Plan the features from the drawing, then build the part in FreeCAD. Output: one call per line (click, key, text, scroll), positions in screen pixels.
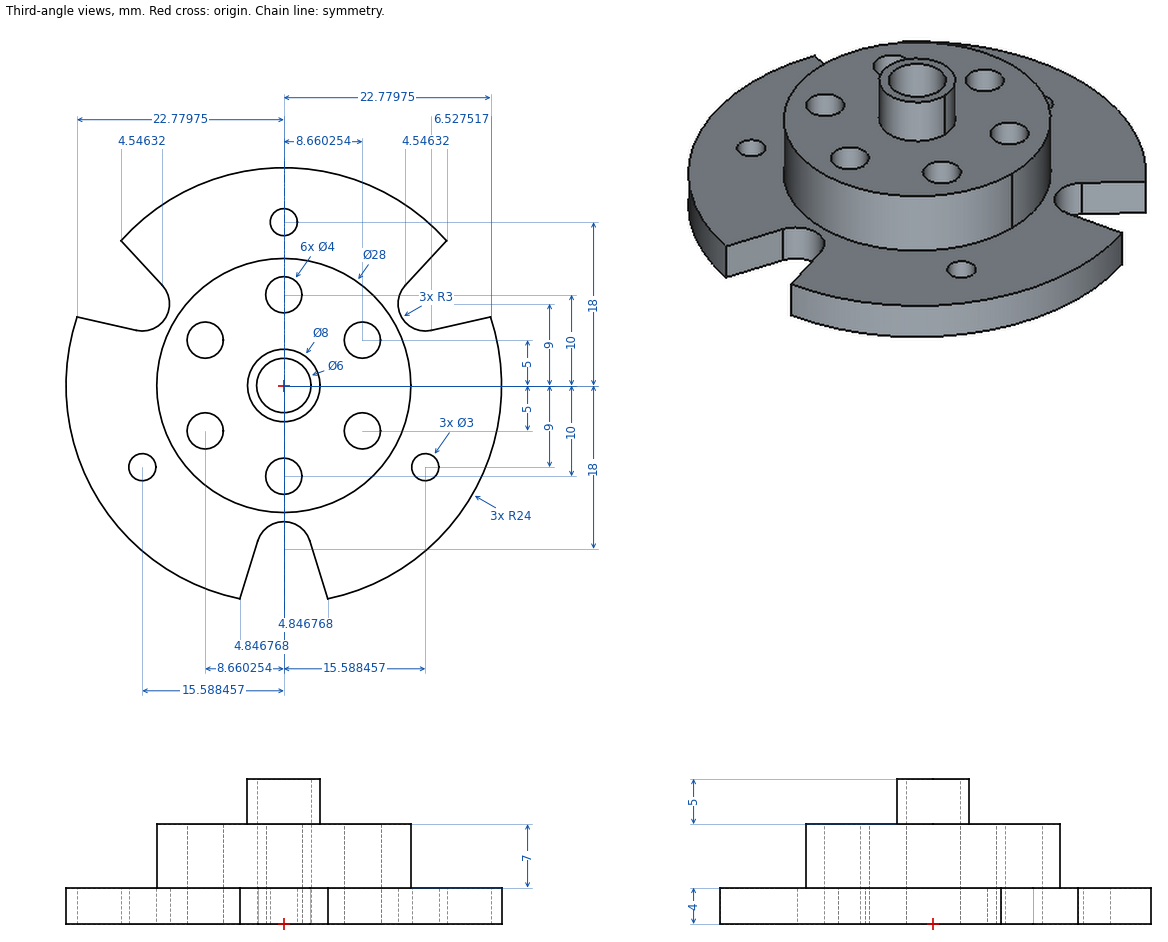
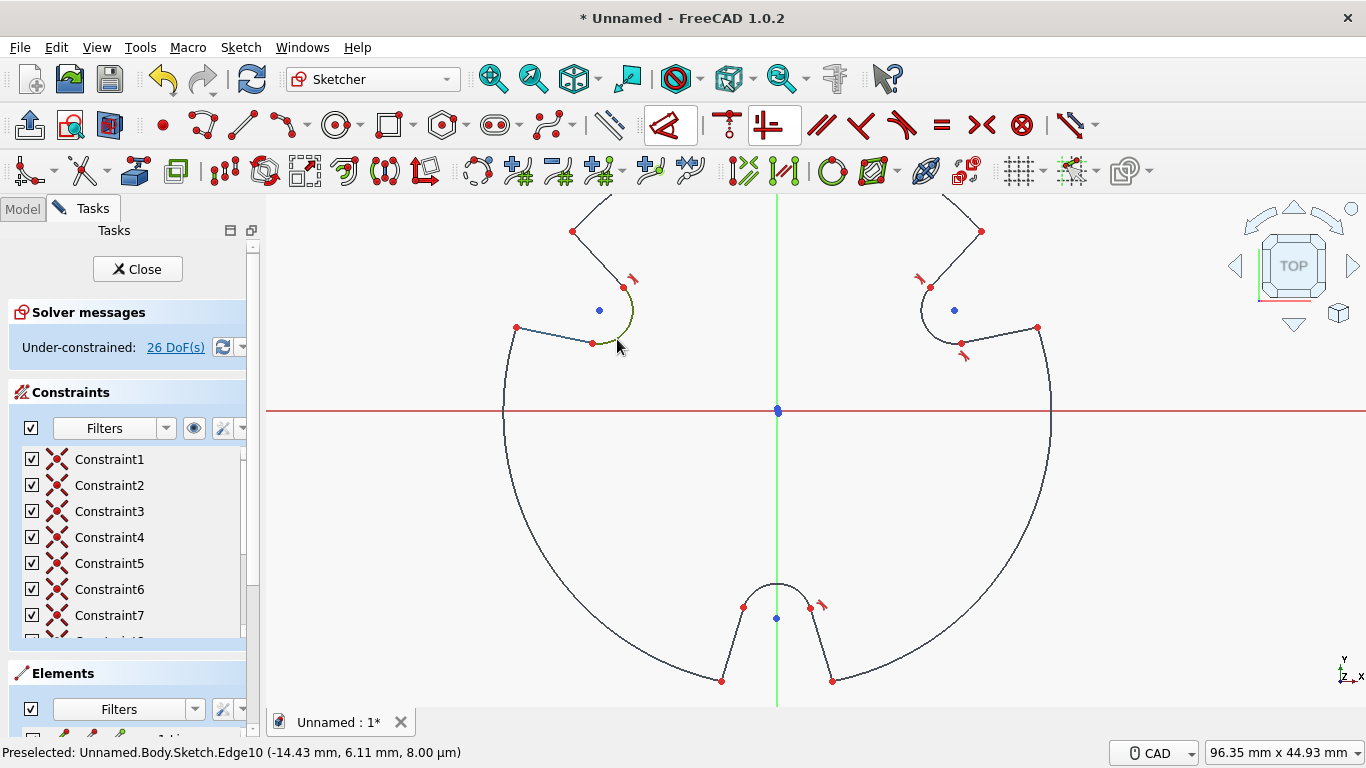
key(t)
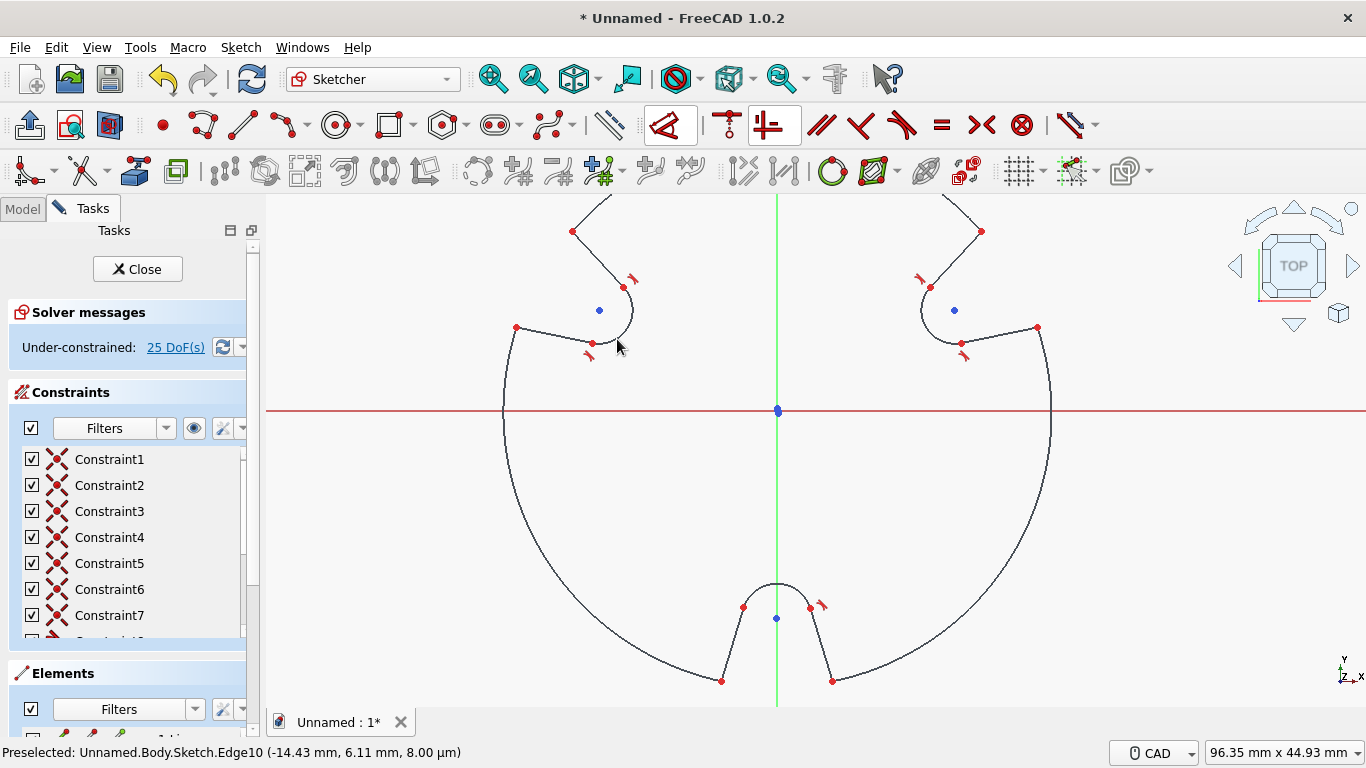
click(728, 659)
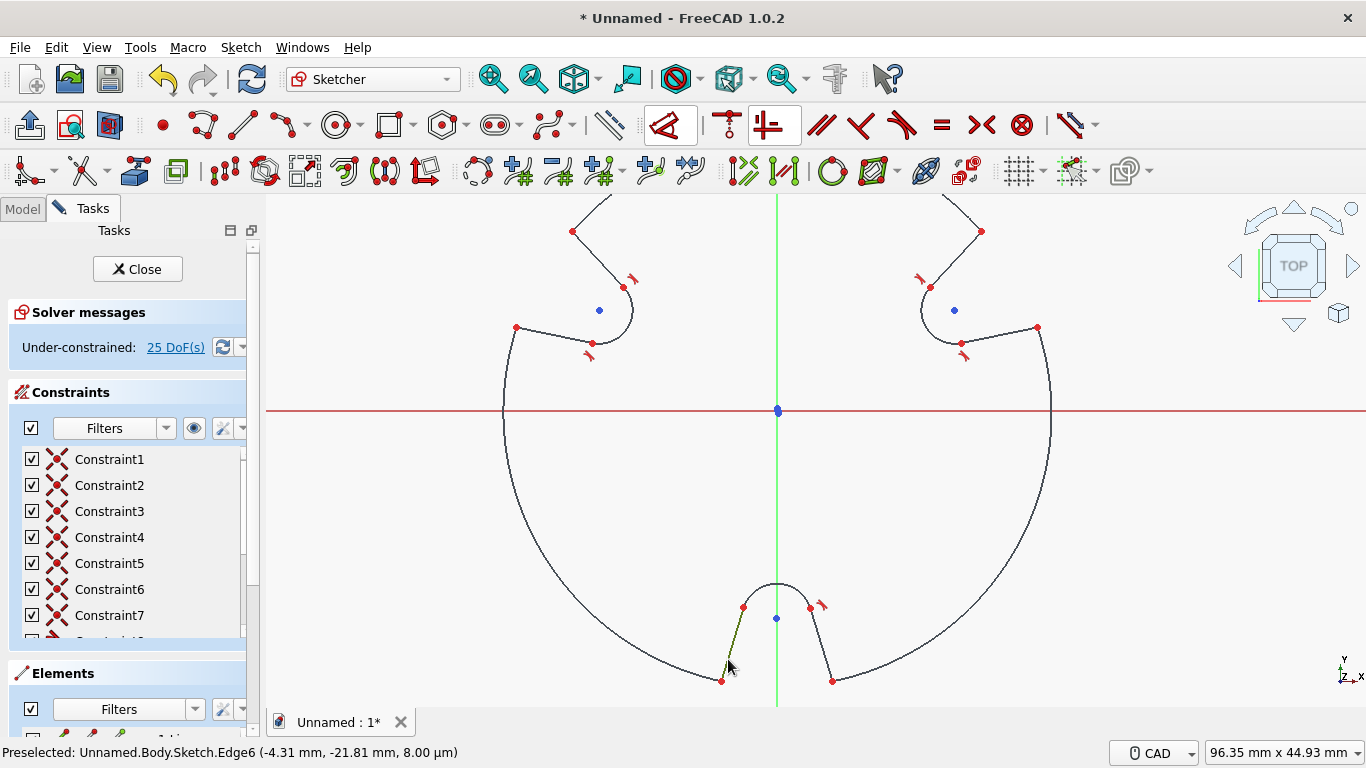
click(794, 588)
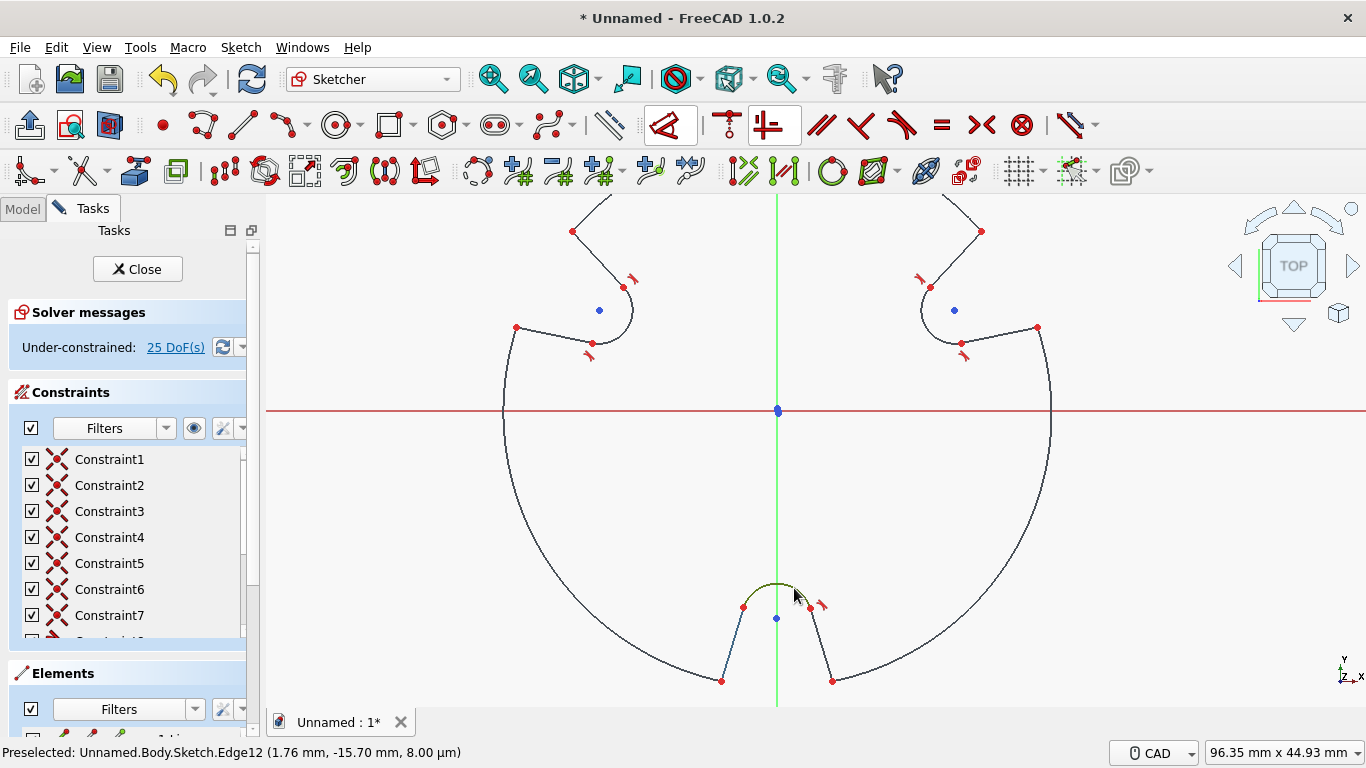
key(t)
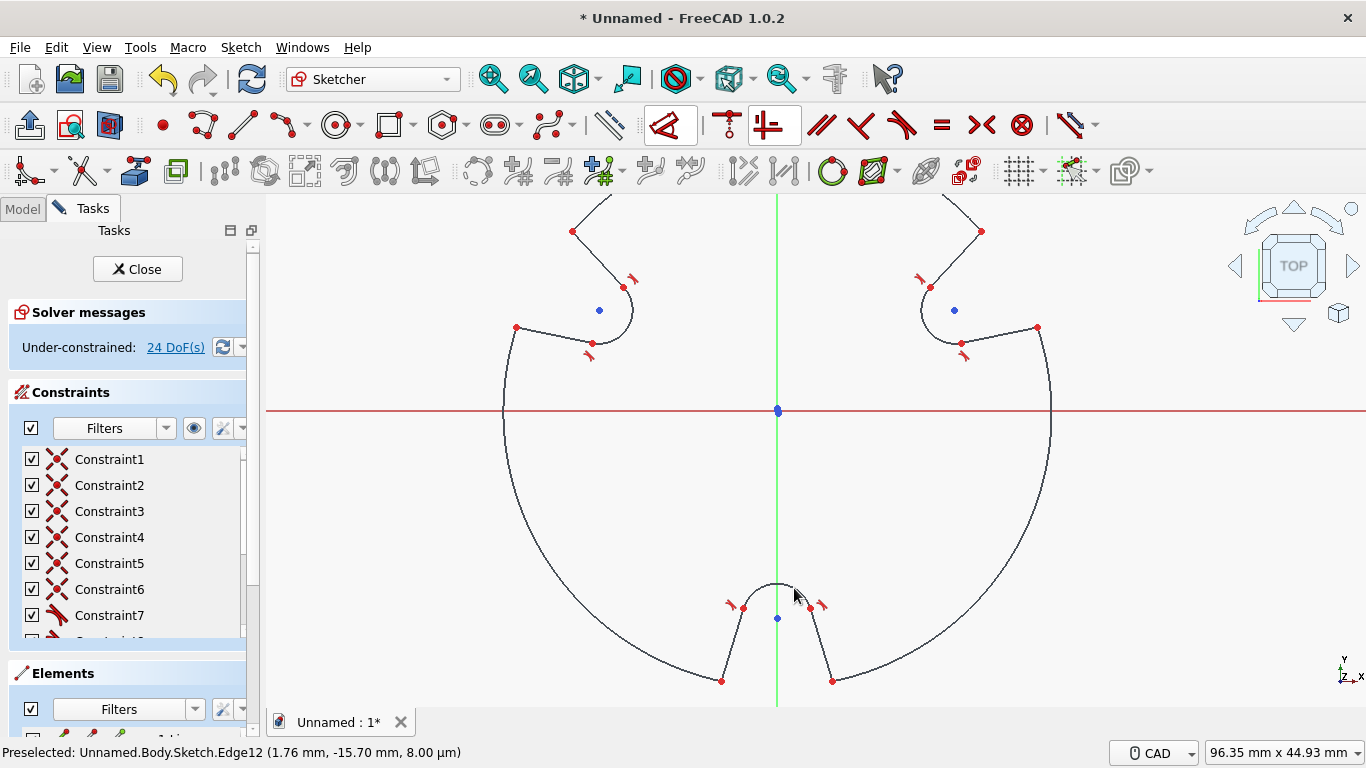
click(956, 621)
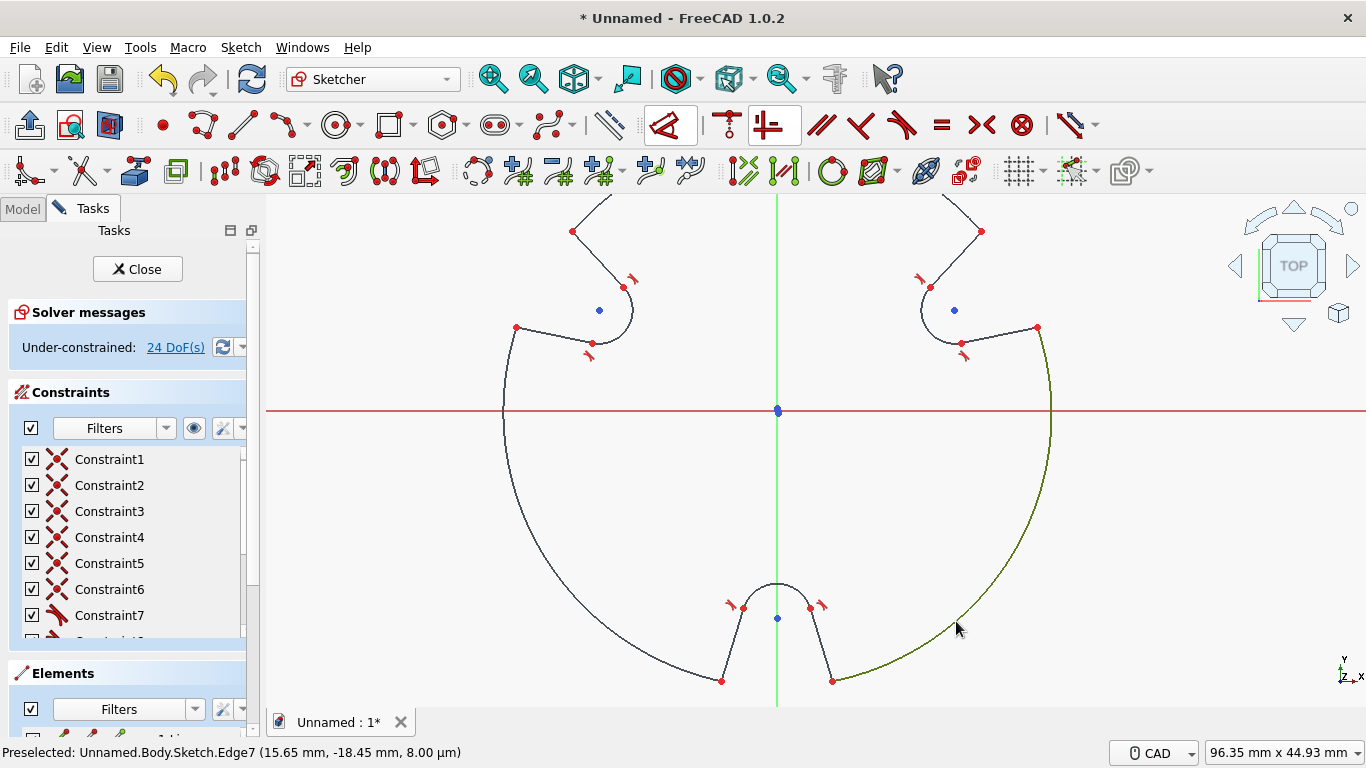
scroll(712, 502, down, 3)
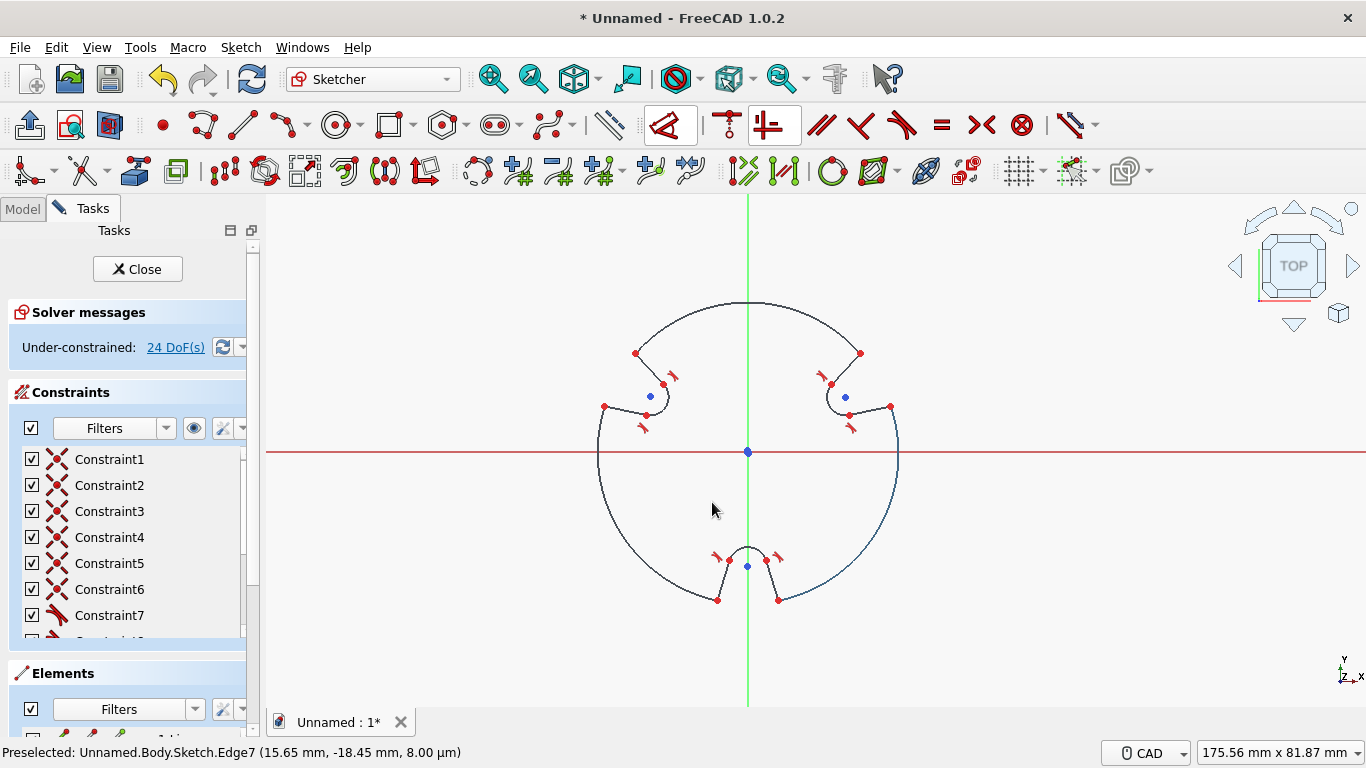
click(798, 311)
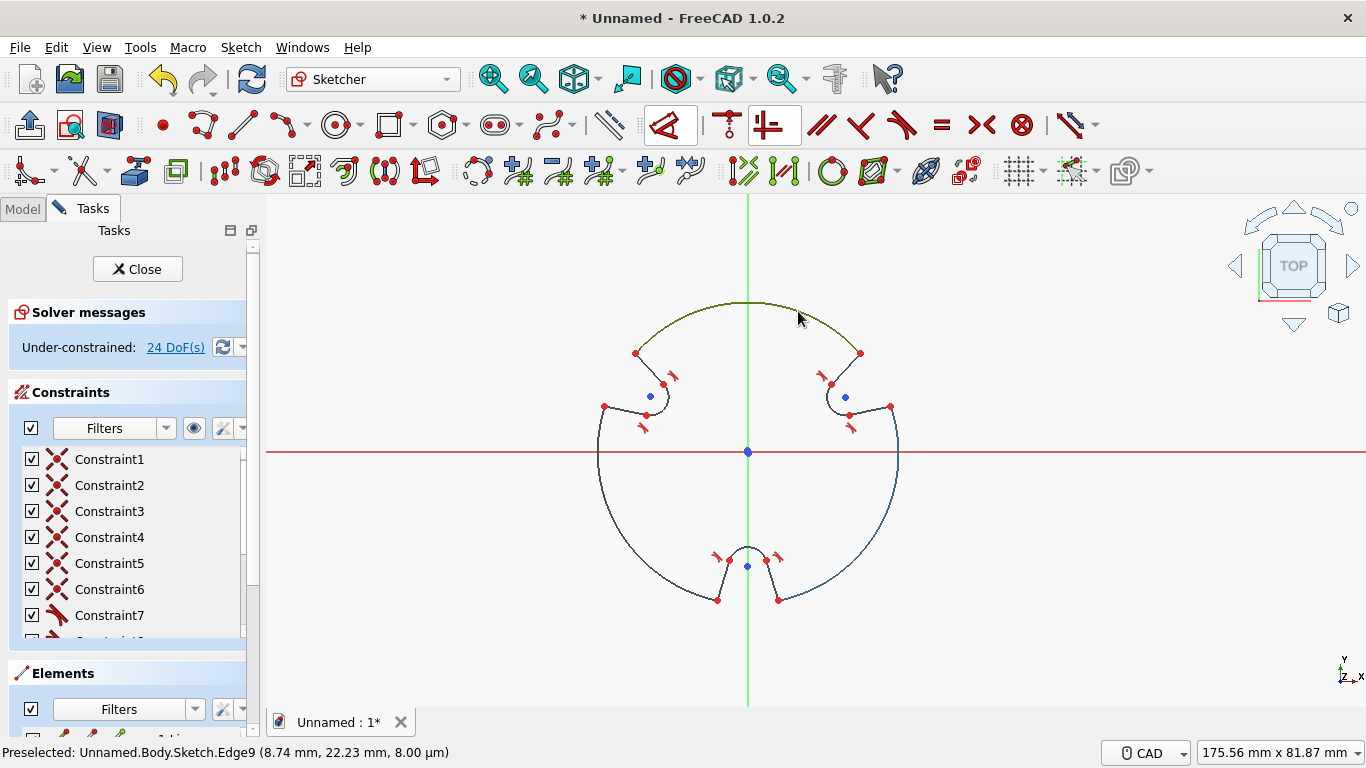
key(c)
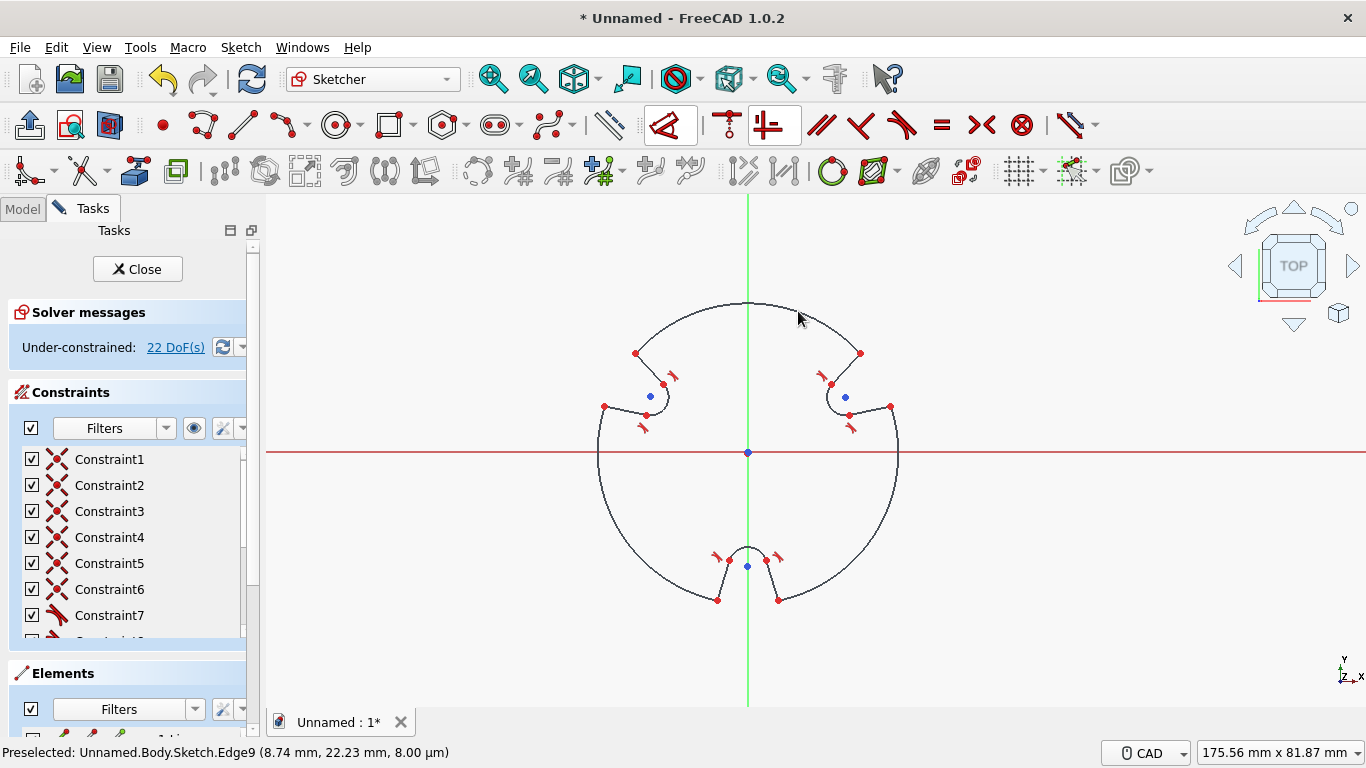
click(846, 568)